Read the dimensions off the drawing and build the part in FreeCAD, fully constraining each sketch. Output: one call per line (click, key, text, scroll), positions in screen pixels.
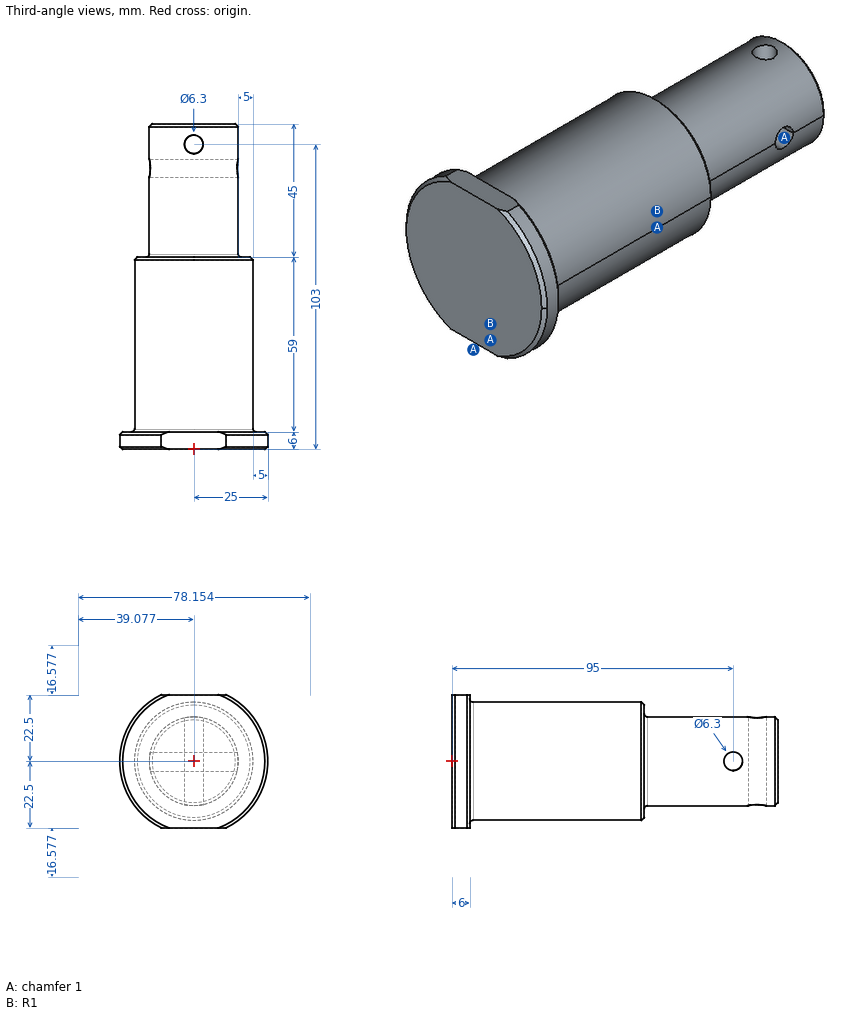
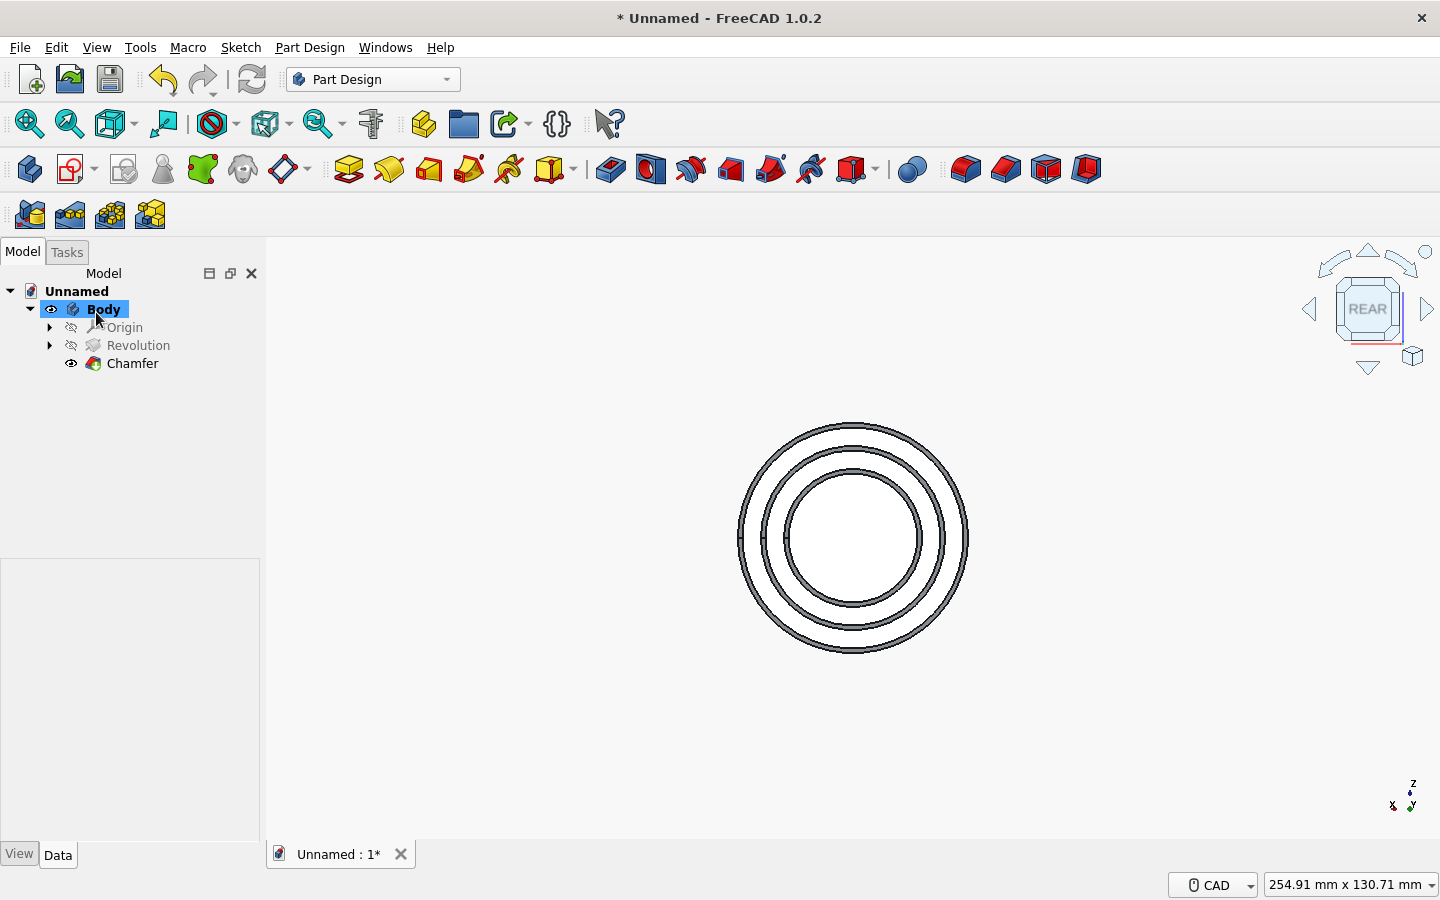
key(6)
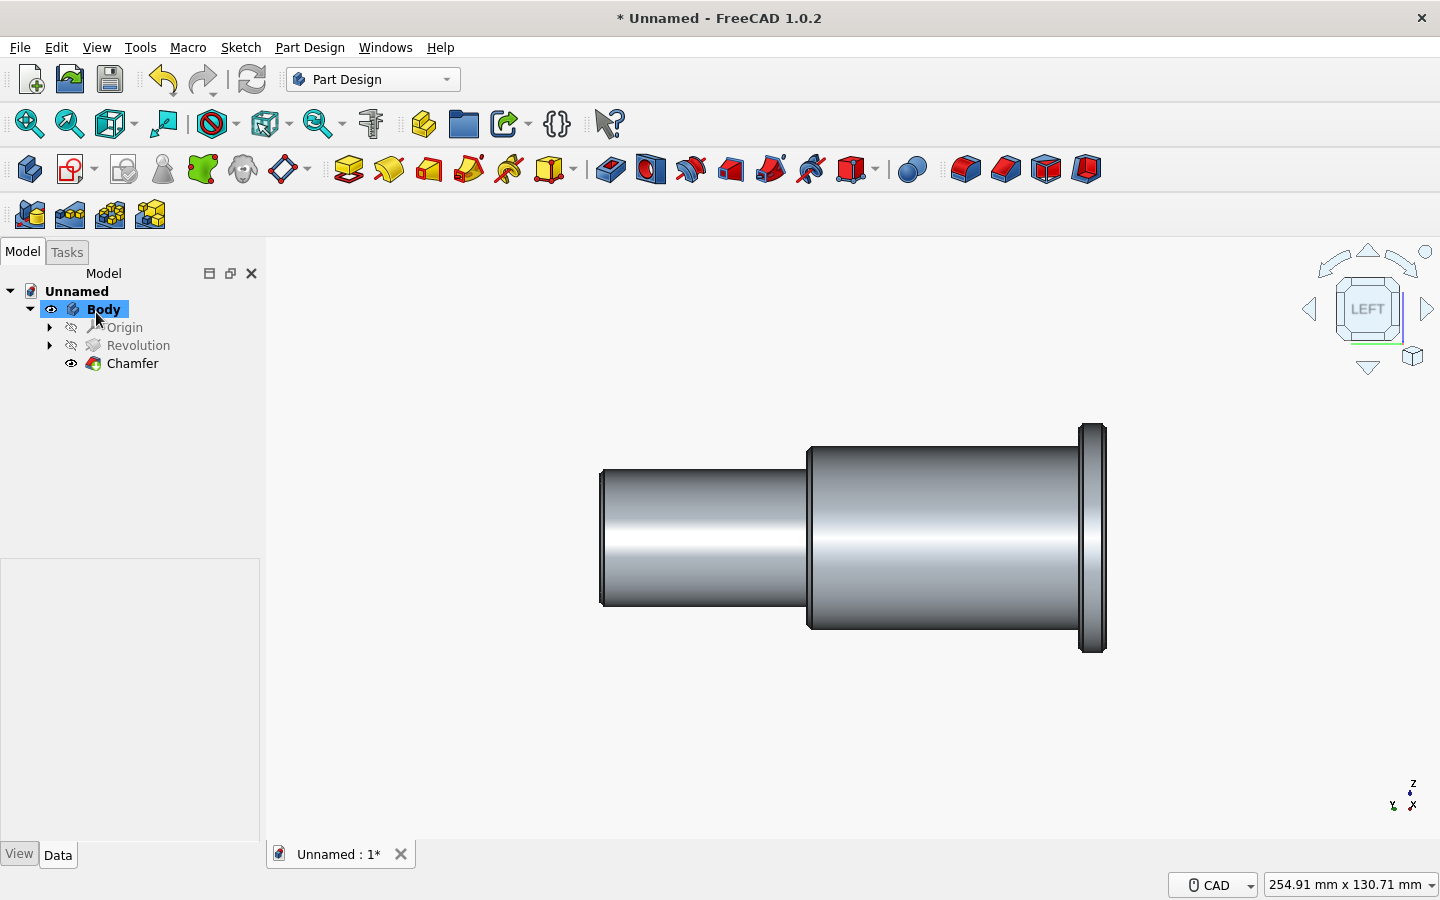
key(v)
key(f)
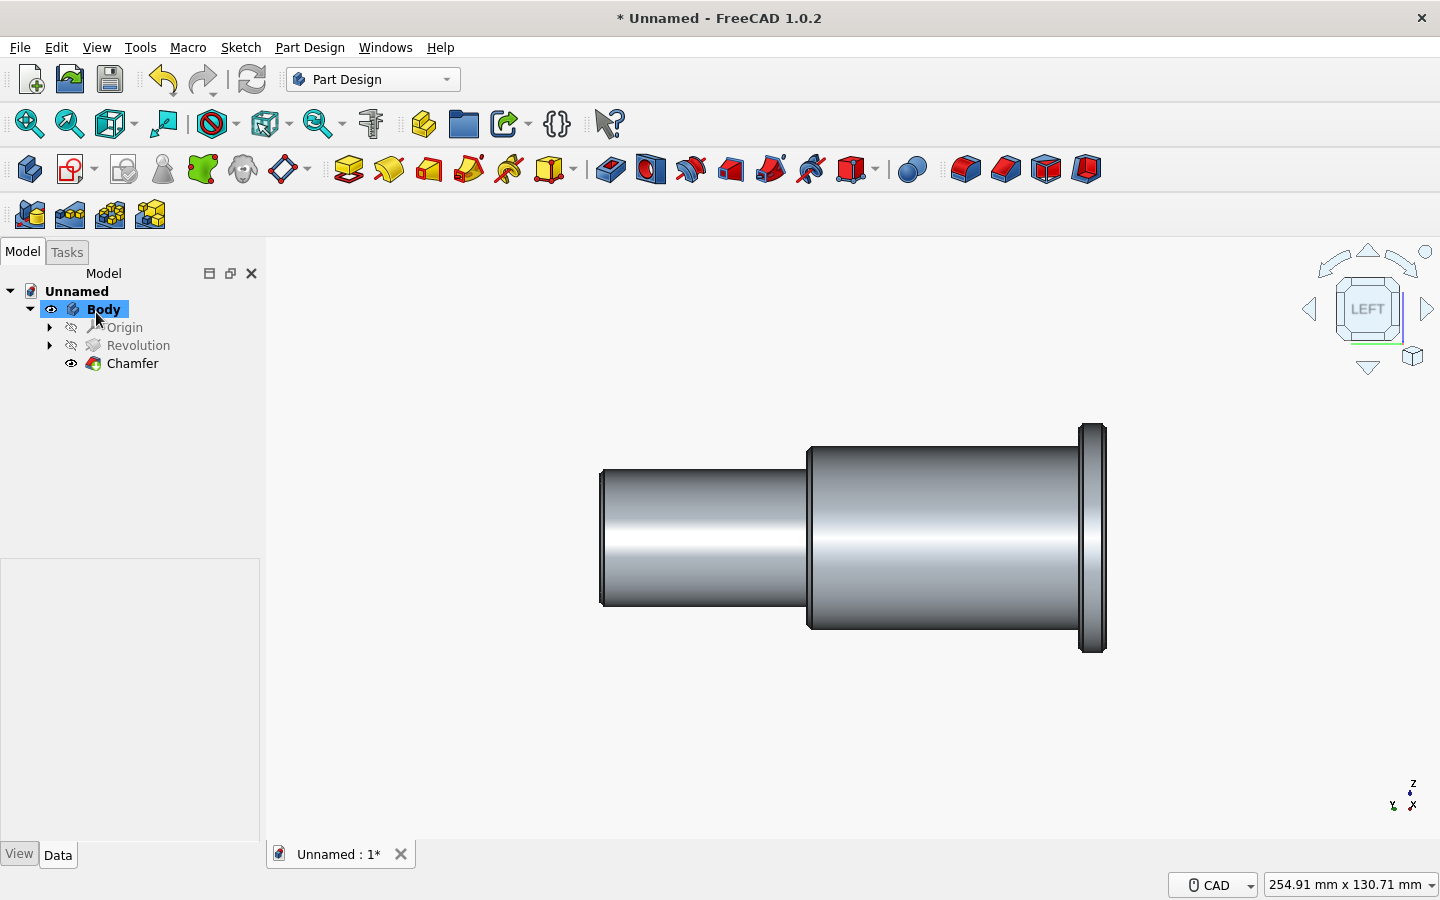
key(v)
key(3)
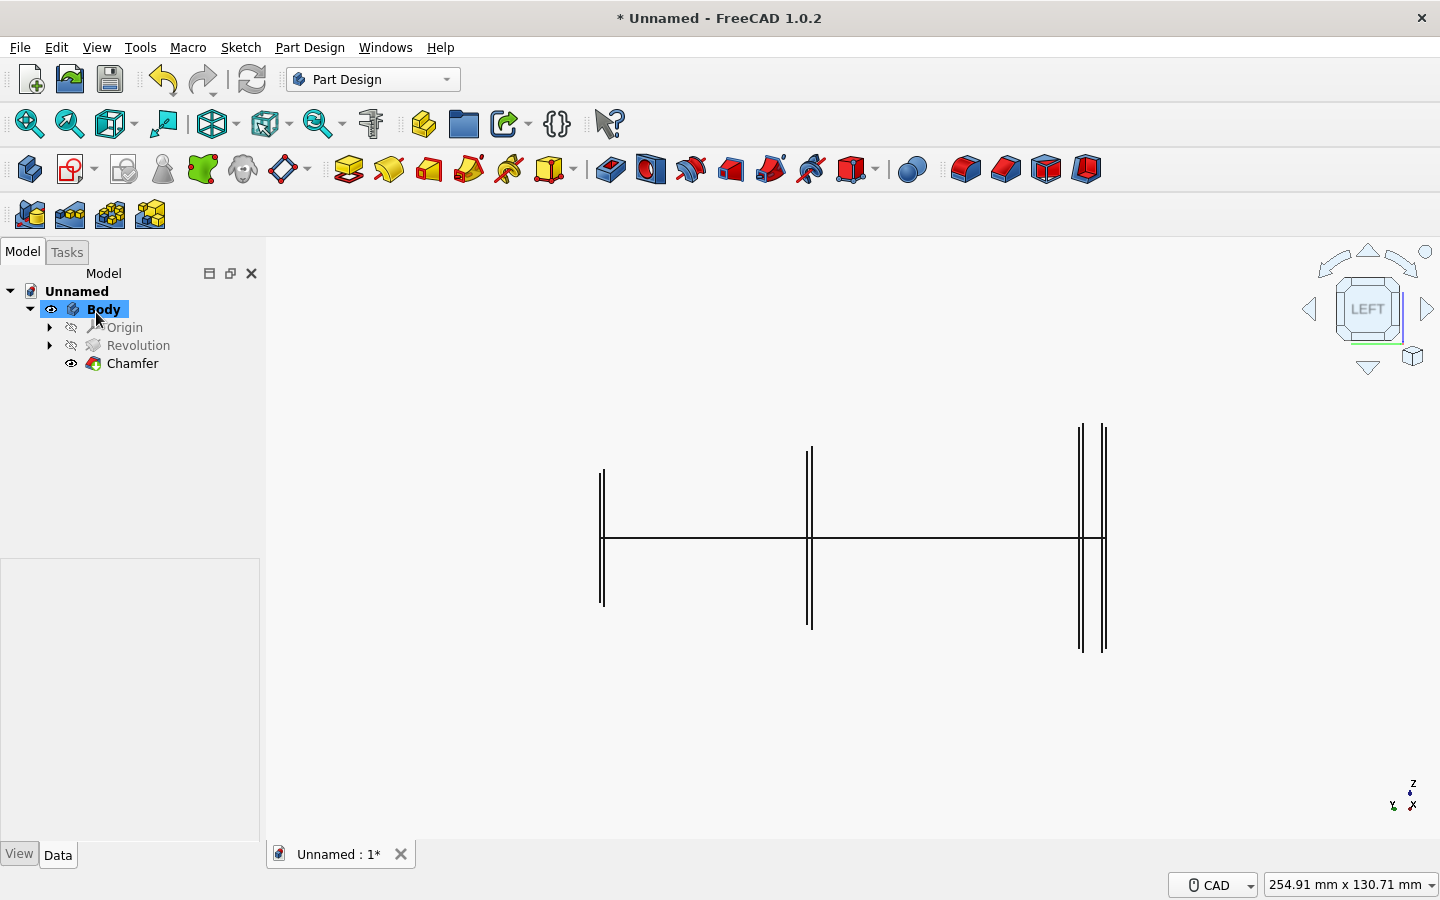
key(0)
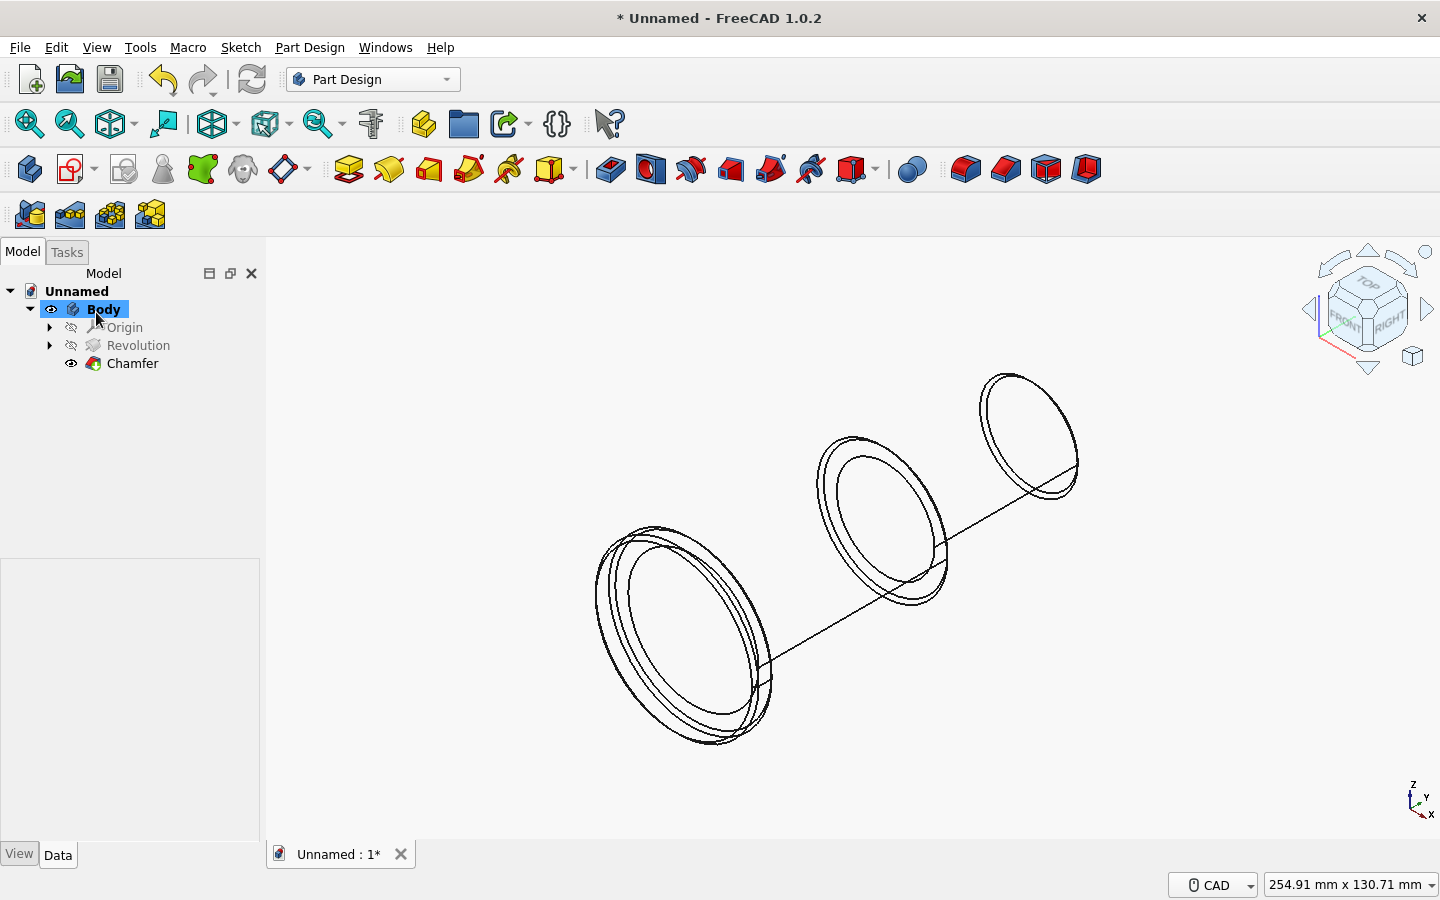
click(837, 490)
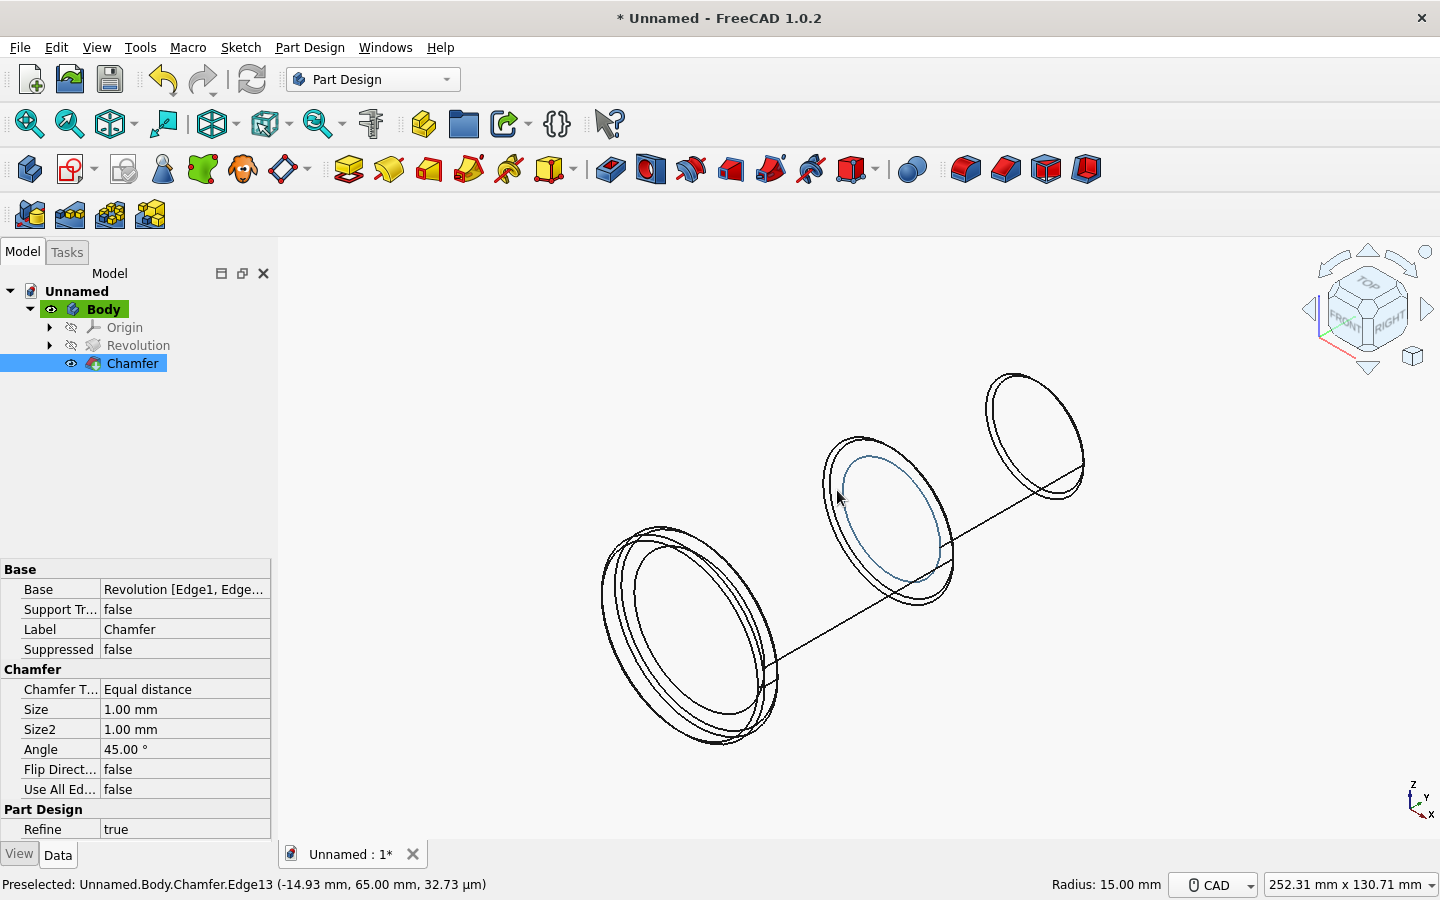
click(634, 592, ctrl)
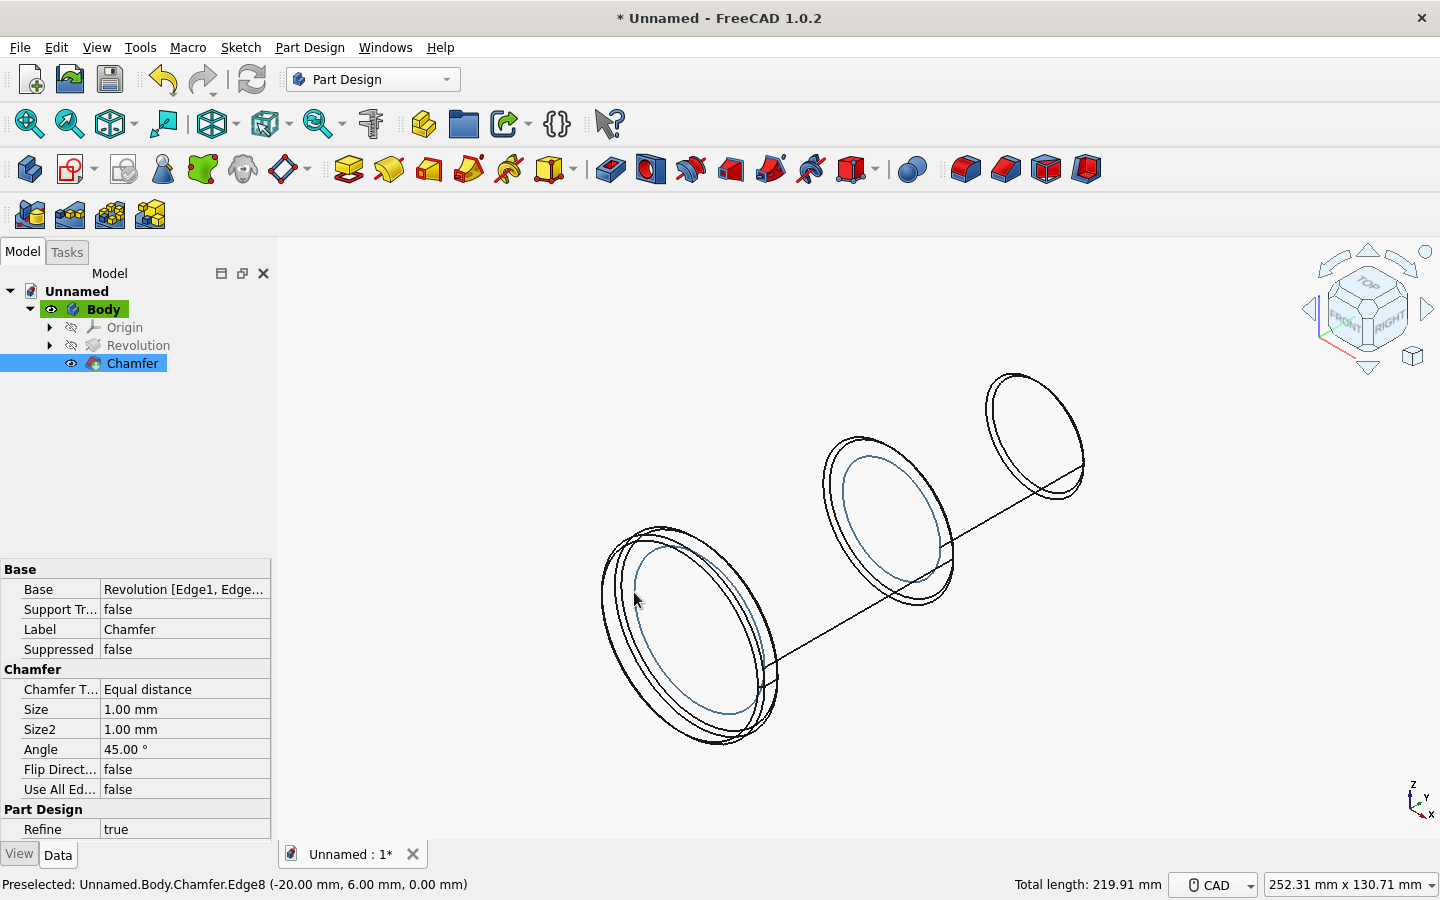
key(v)
key(1)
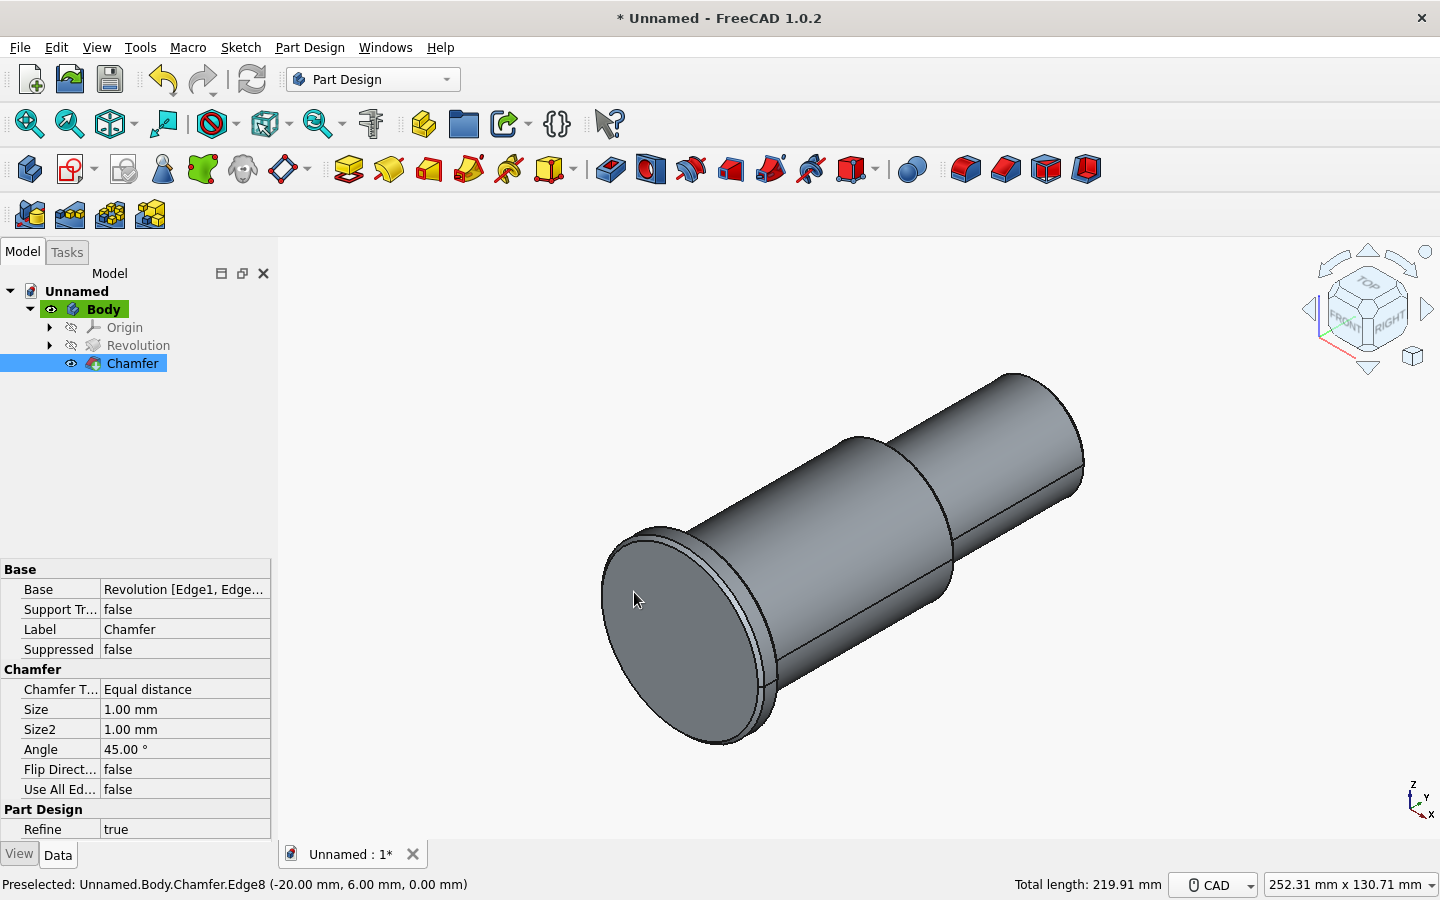
click(966, 170)